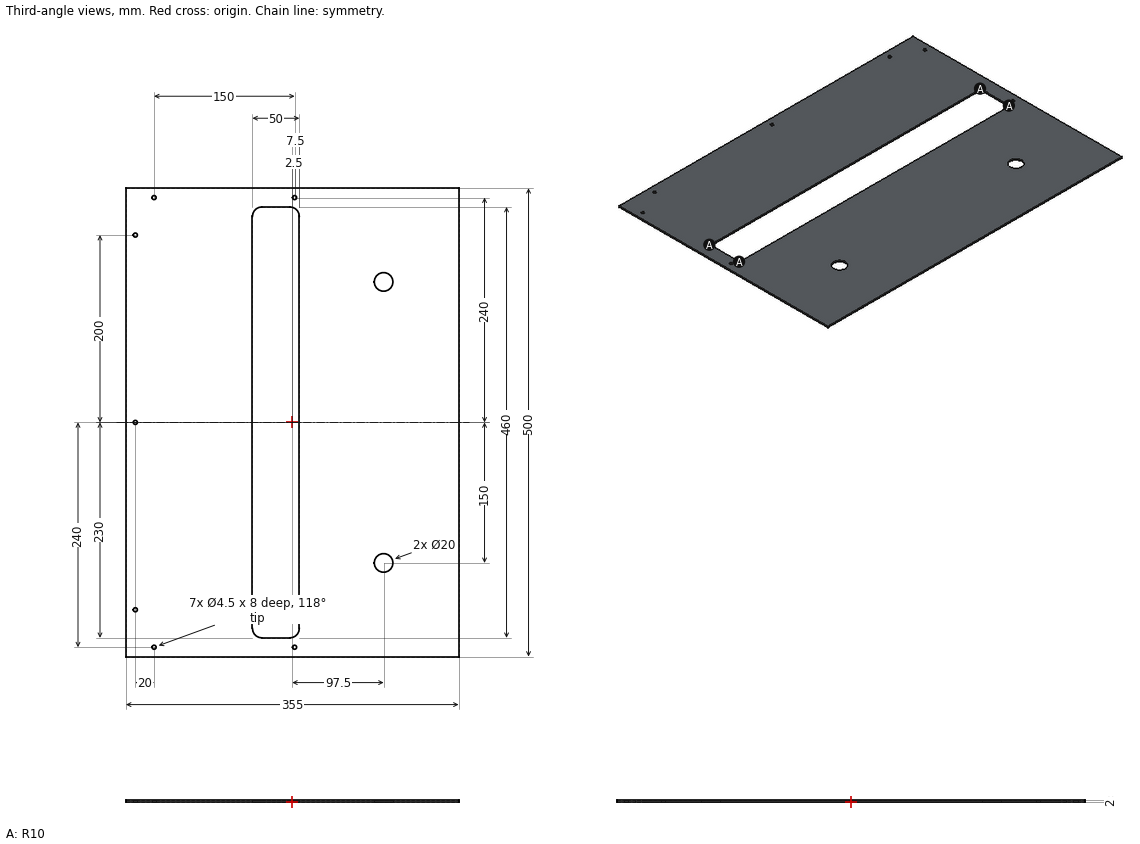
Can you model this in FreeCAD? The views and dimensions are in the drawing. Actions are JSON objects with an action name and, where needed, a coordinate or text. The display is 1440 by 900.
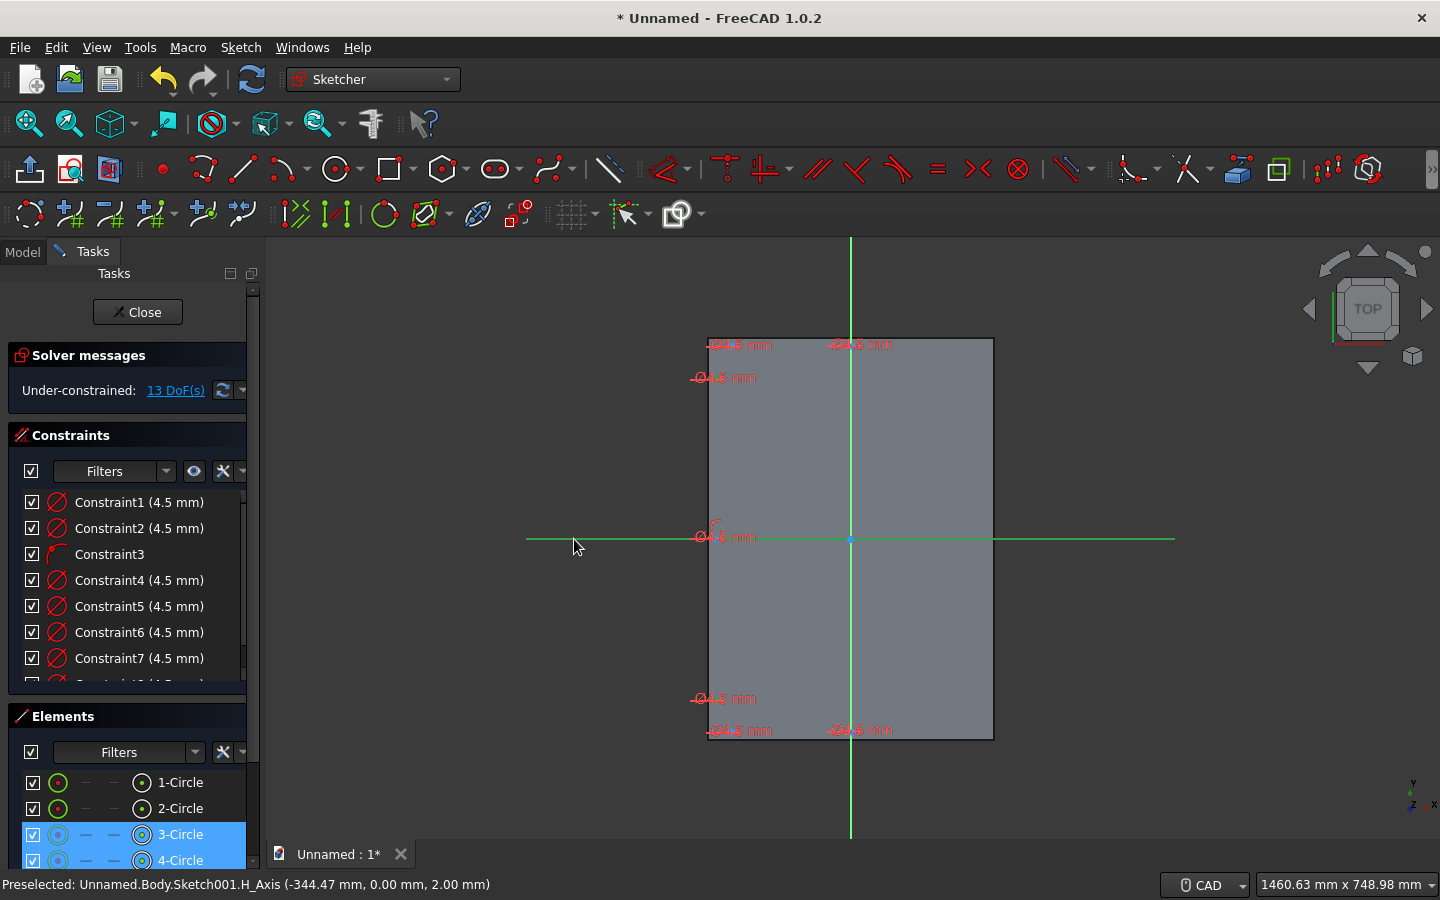
{"action": "key", "text": "s"}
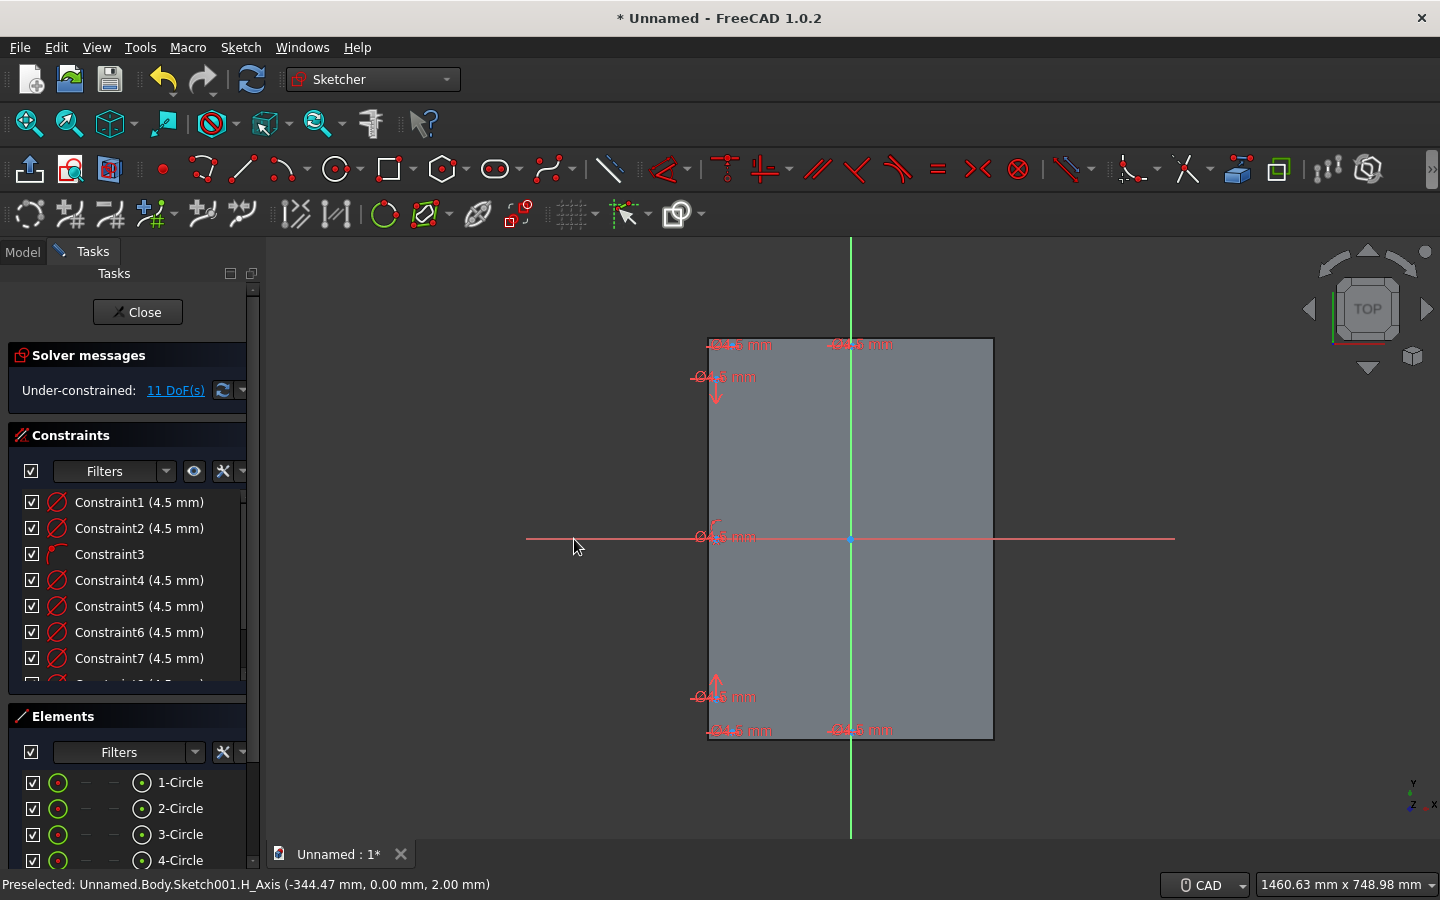
{"action": "left_click", "coordinate": [732, 733]}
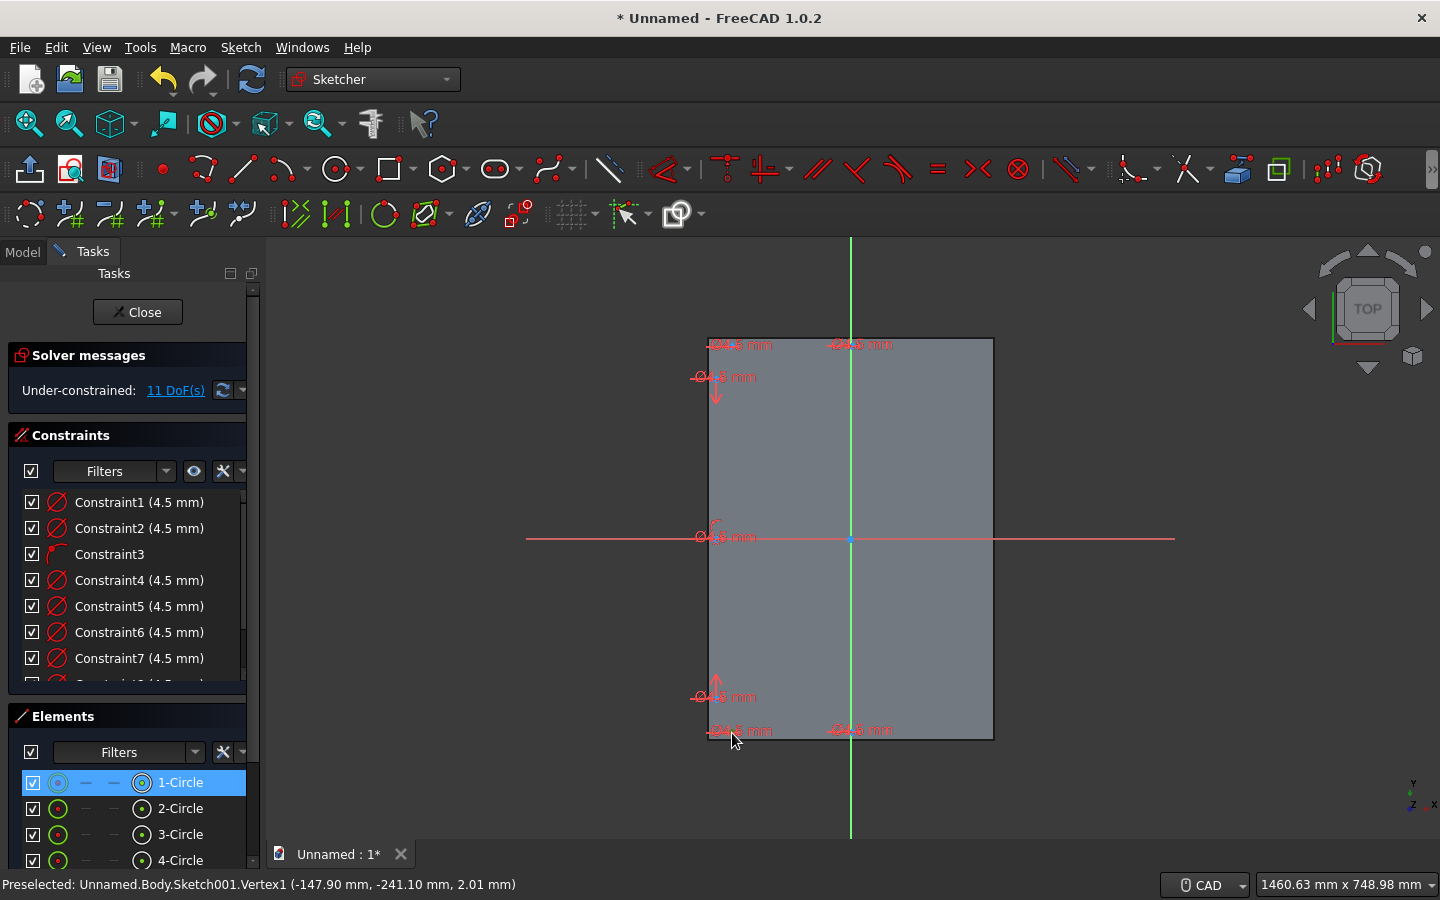
{"action": "left_click", "coordinate": [732, 347]}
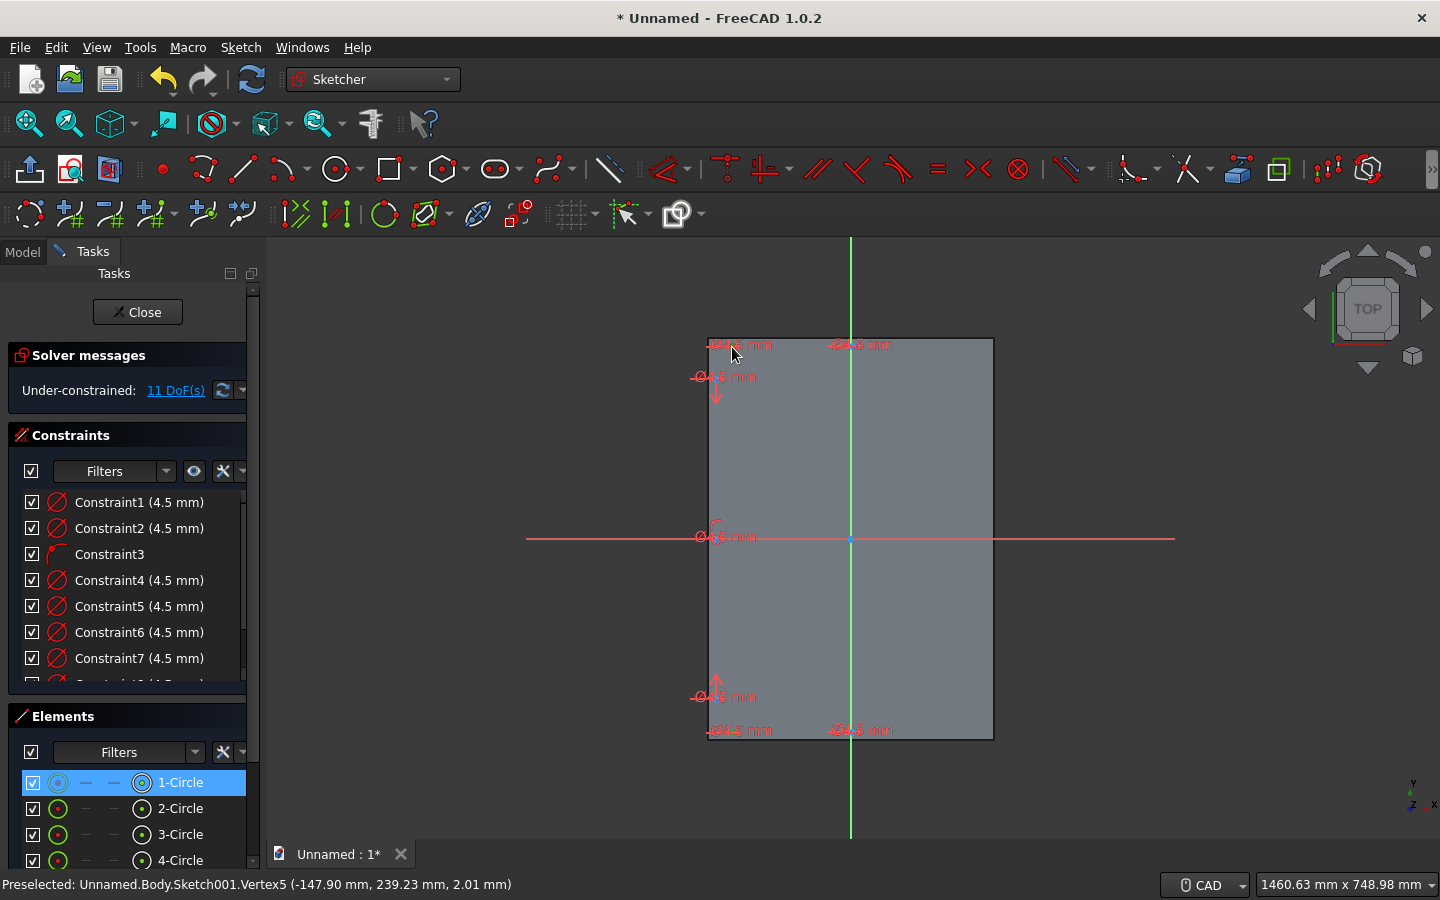
{"action": "left_click", "coordinate": [574, 539]}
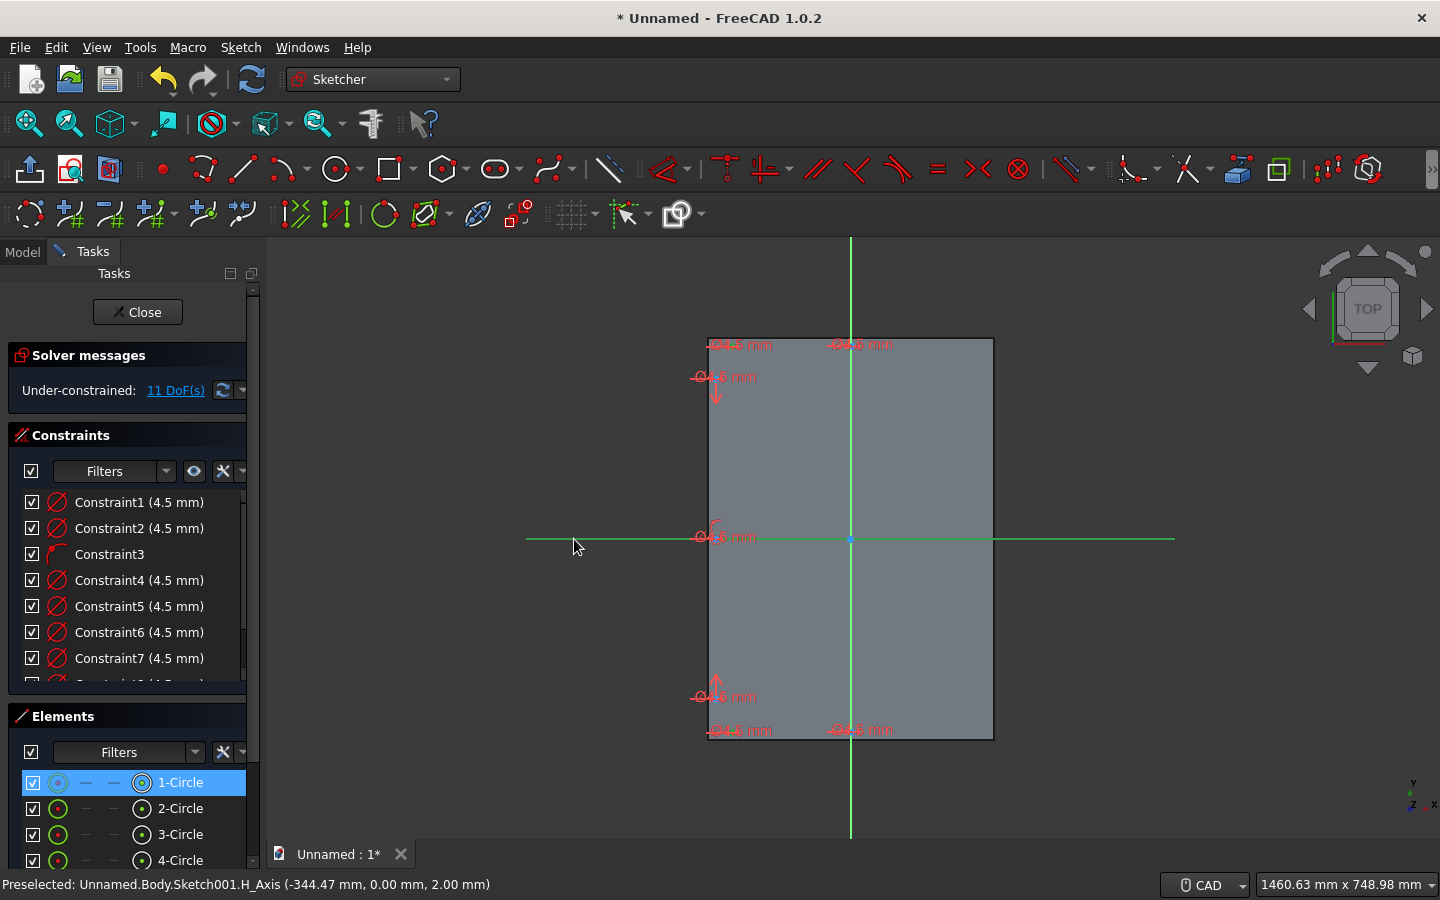
{"action": "key", "text": "s"}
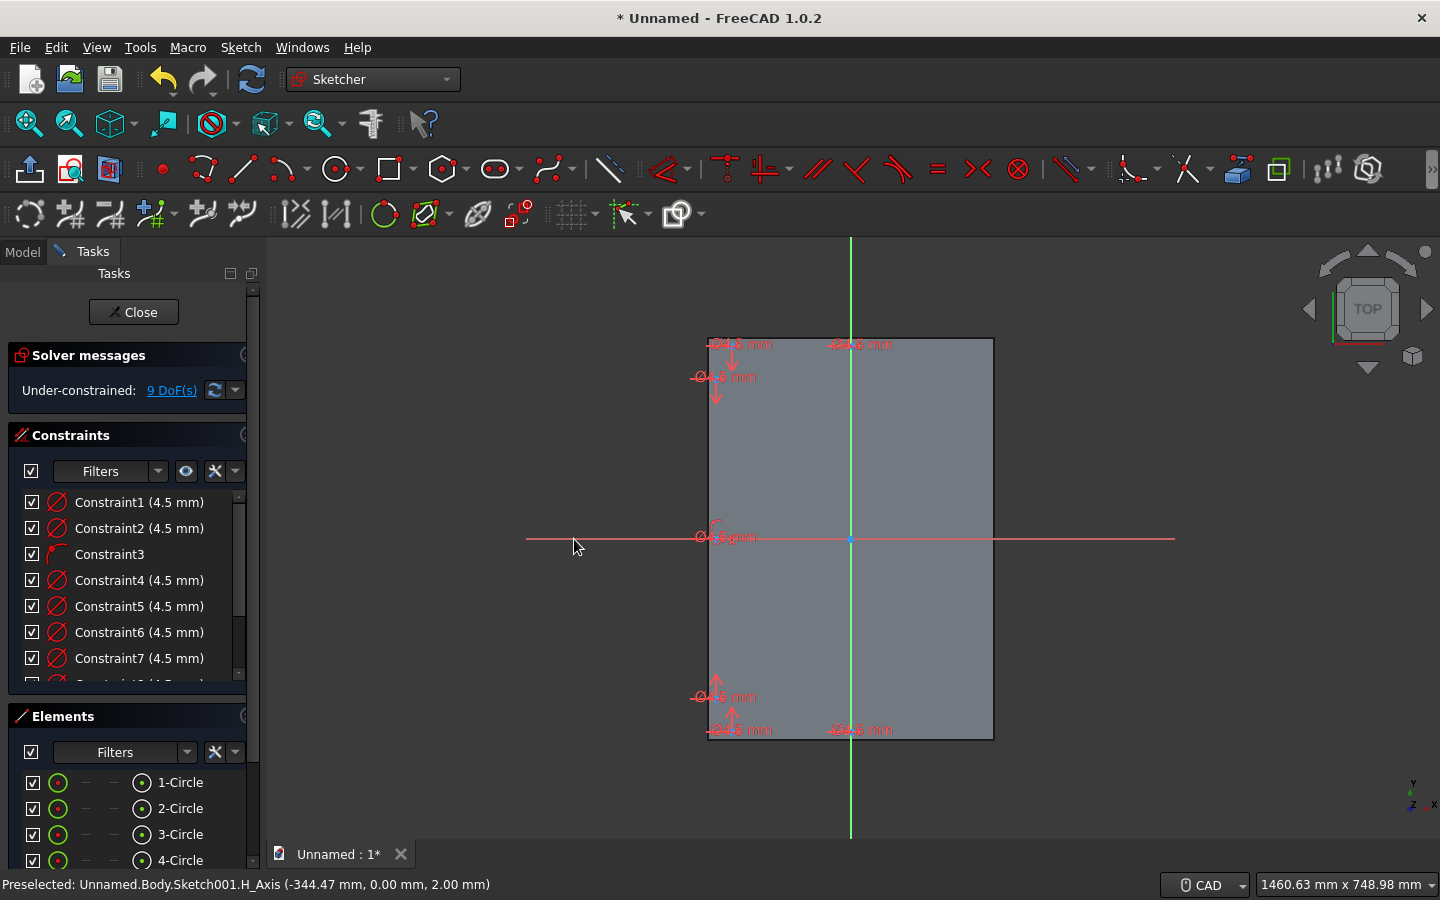
{"action": "left_click", "coordinate": [853, 346]}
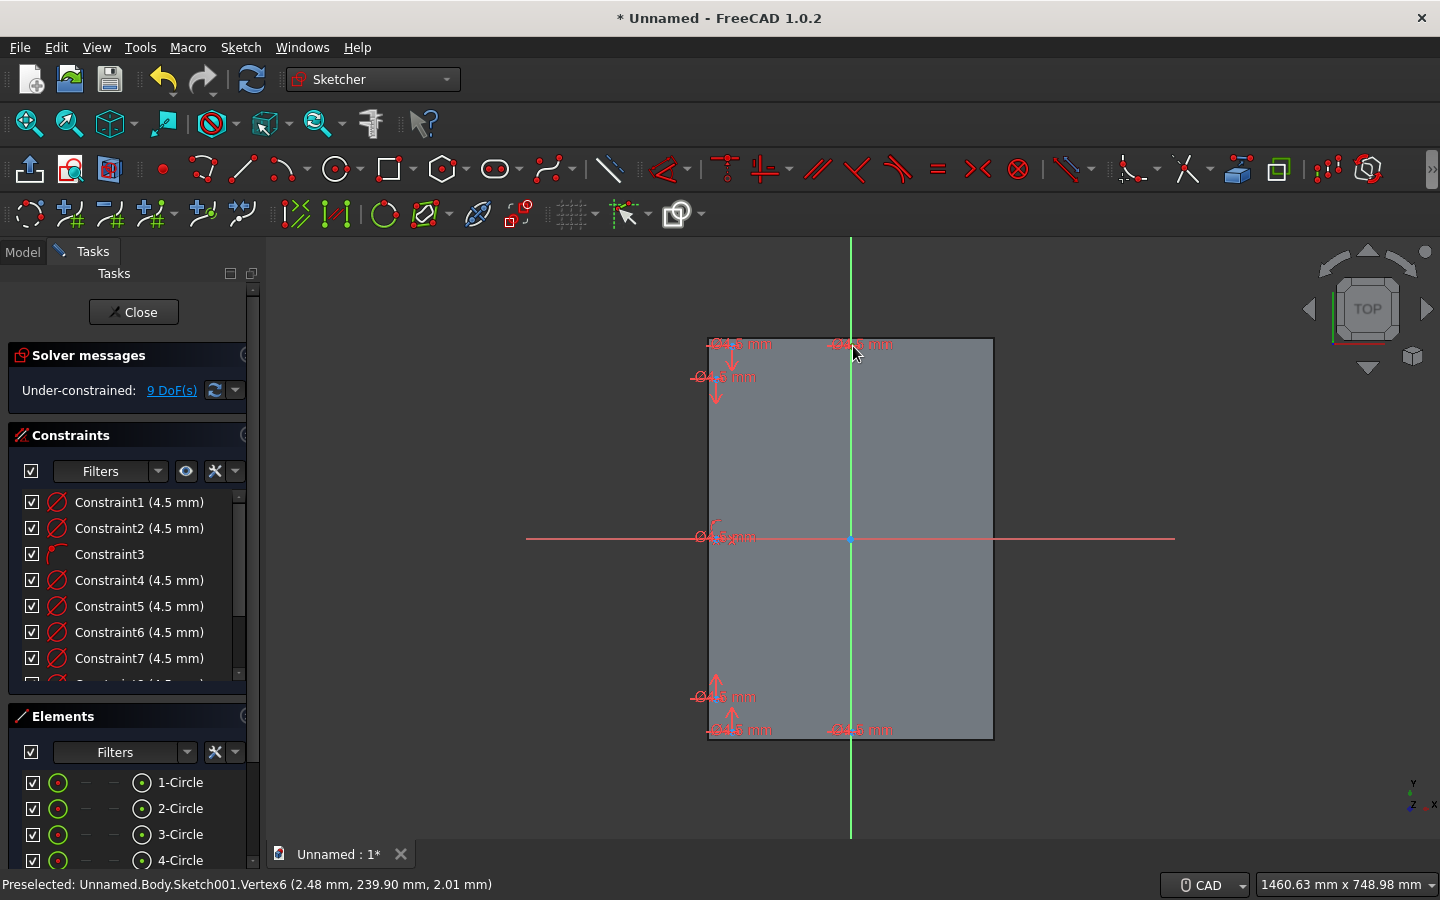
{"action": "left_click", "coordinate": [853, 732]}